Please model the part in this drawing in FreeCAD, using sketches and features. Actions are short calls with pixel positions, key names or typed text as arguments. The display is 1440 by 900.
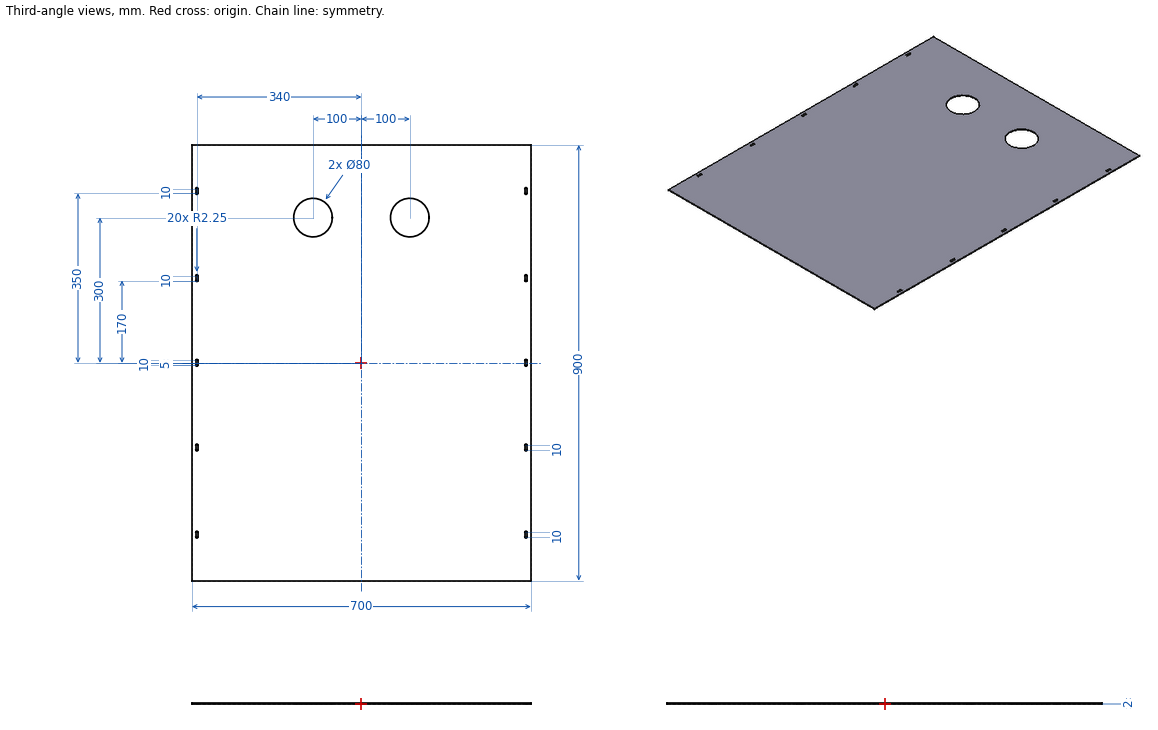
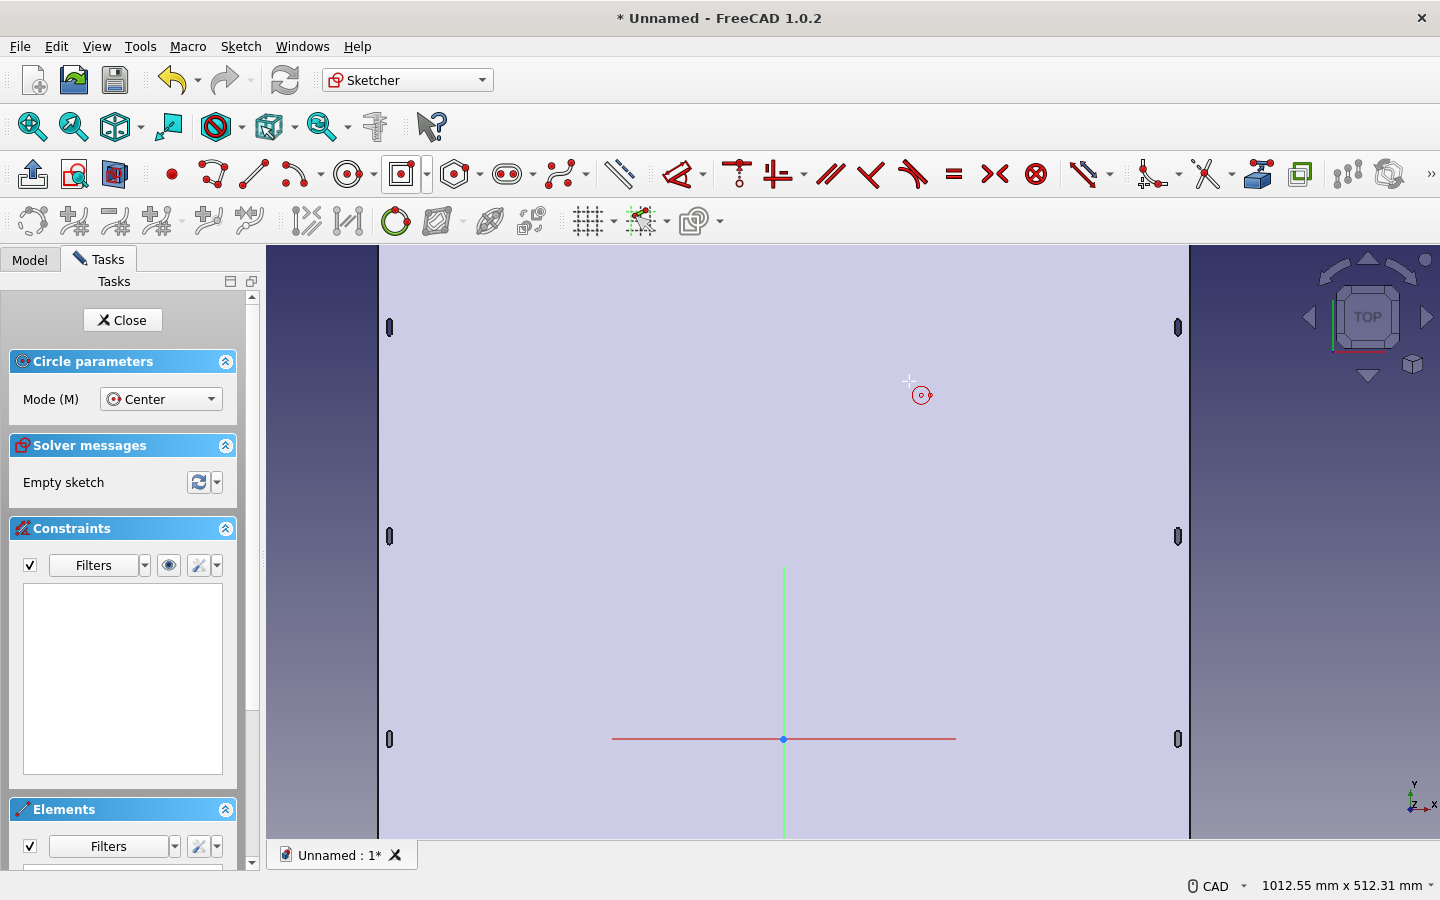
click(668, 391)
click(701, 358)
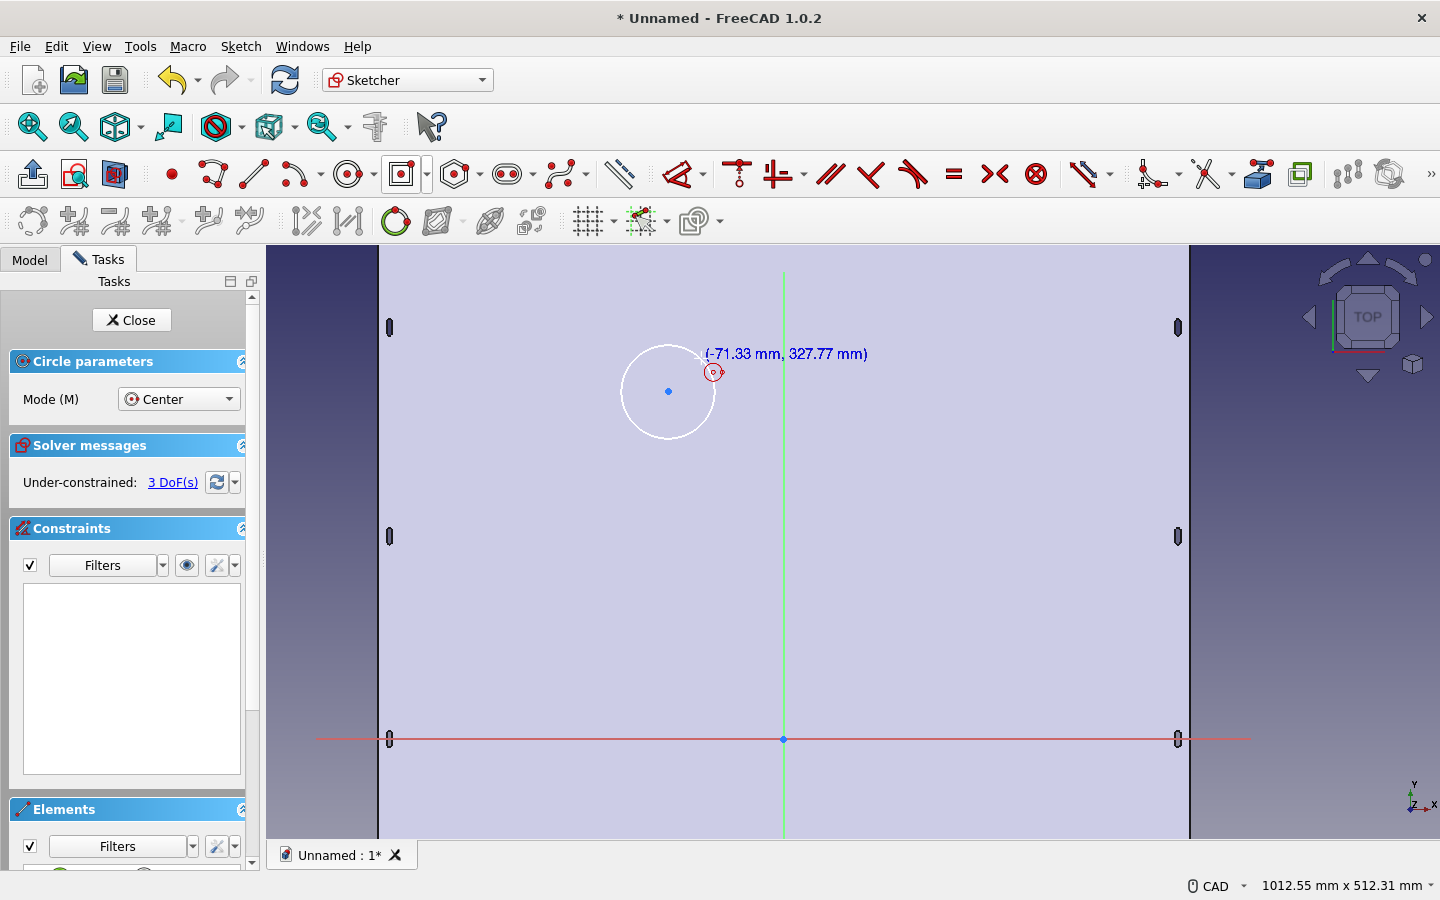
click(900, 391)
click(932, 358)
key(Escape)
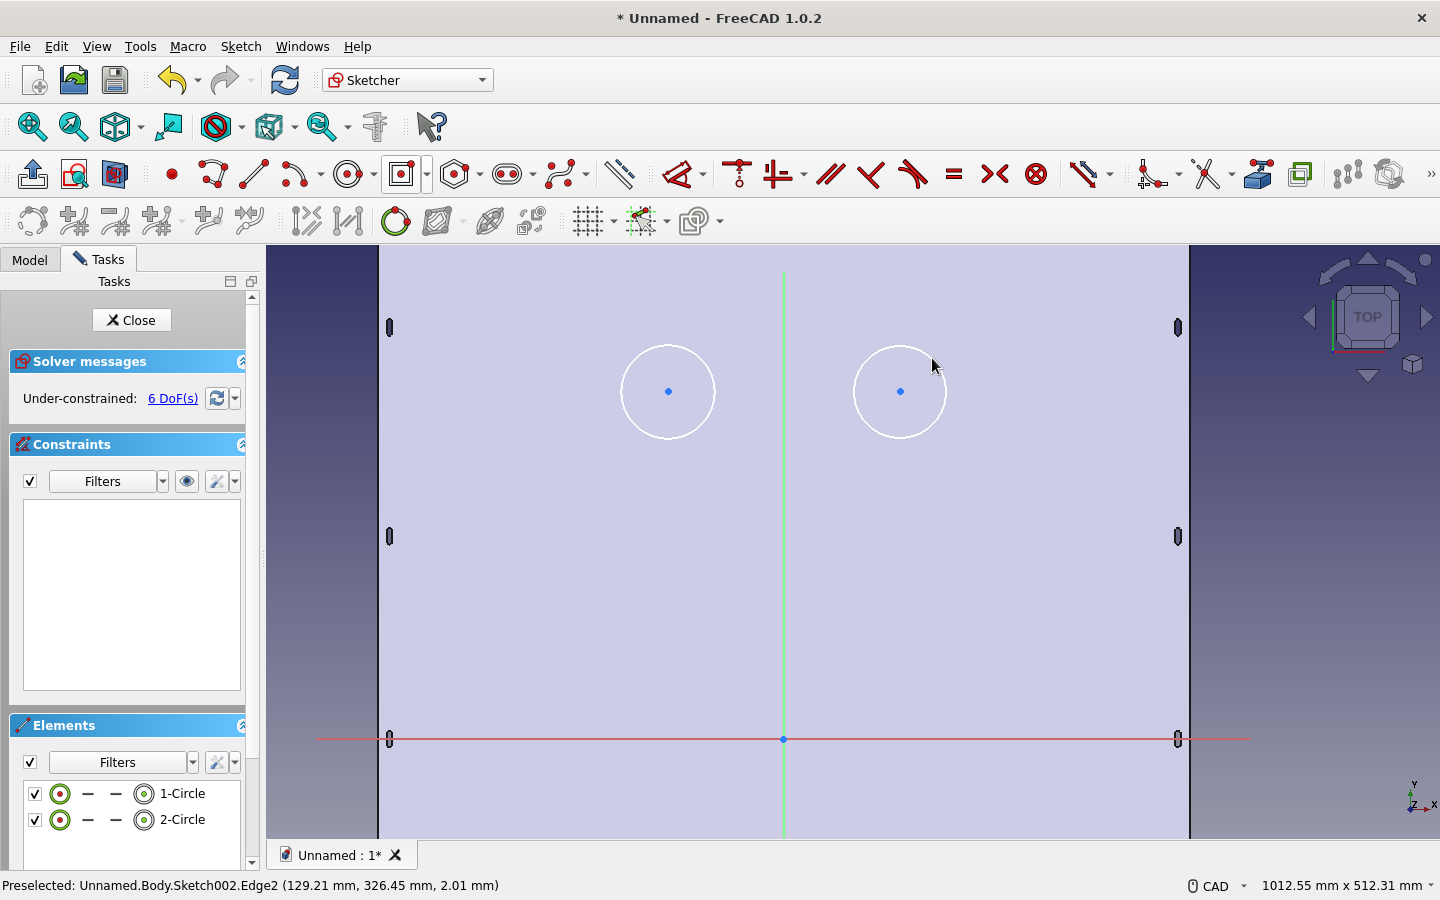
click(701, 359)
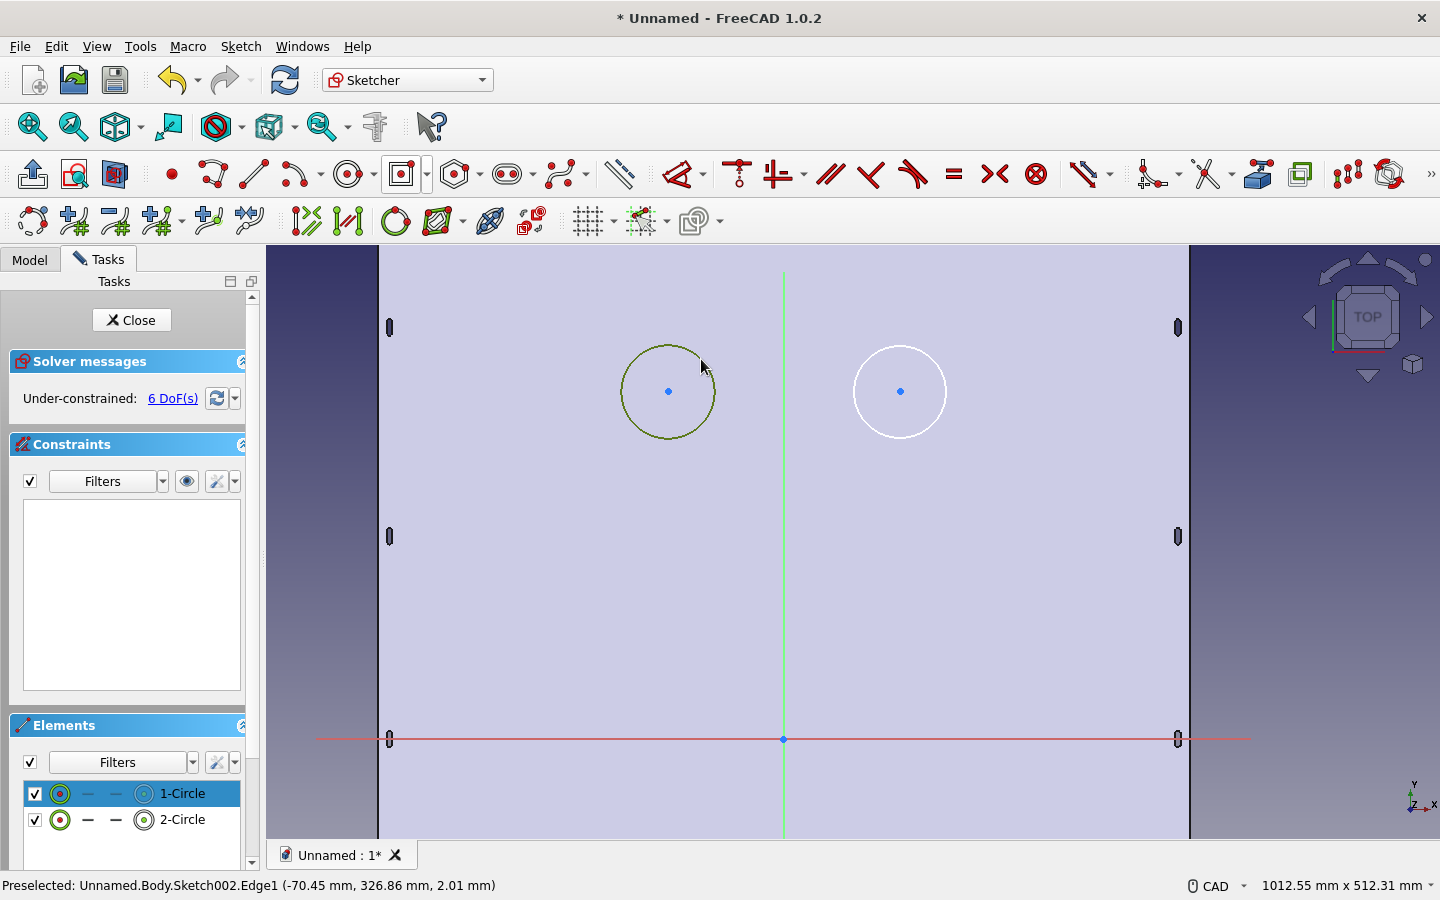
click(932, 359)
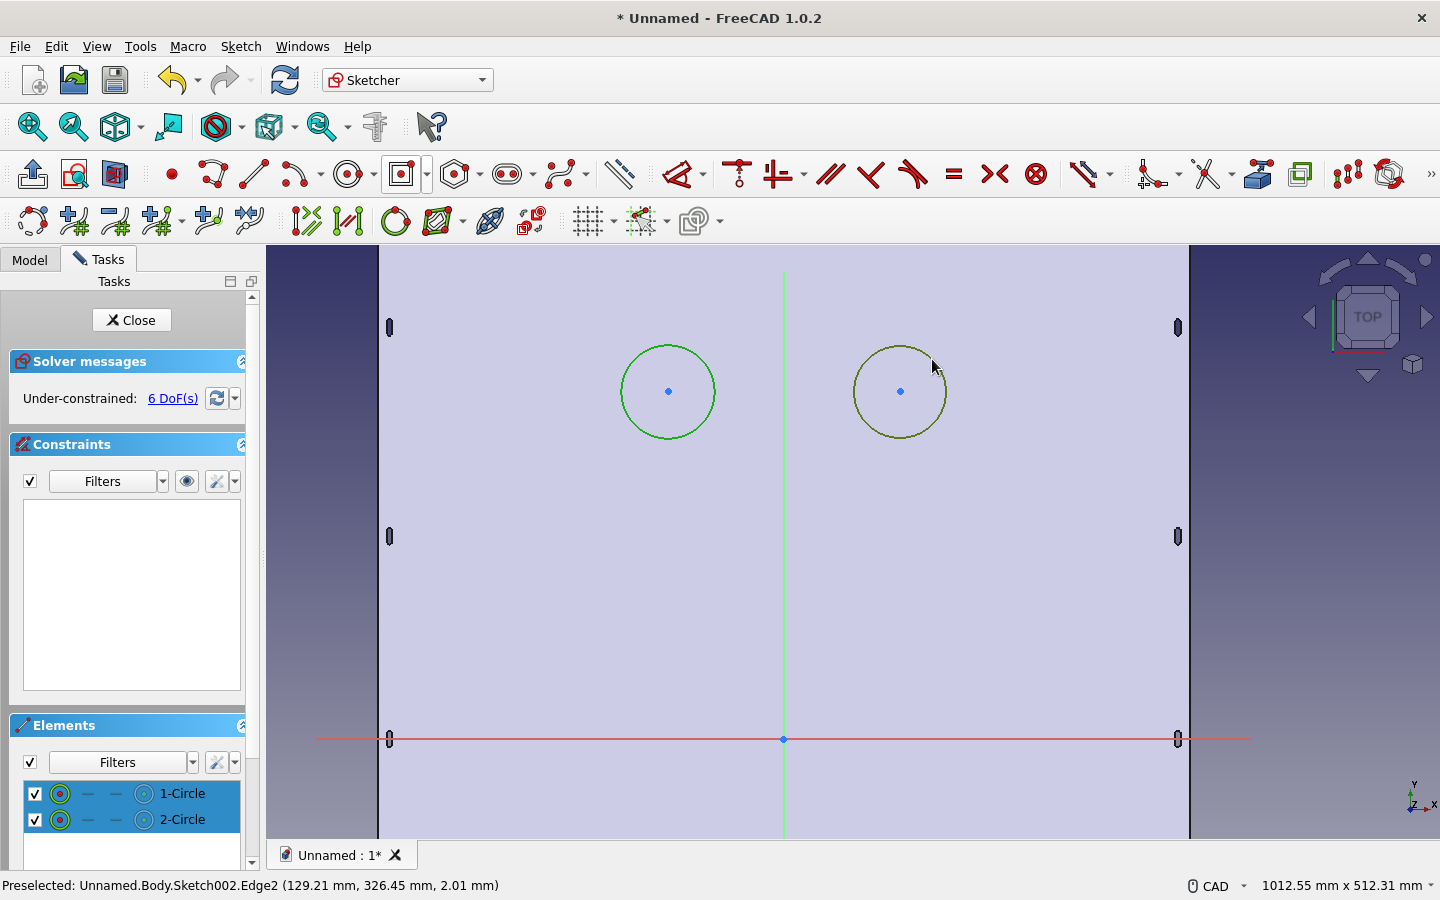
click(954, 174)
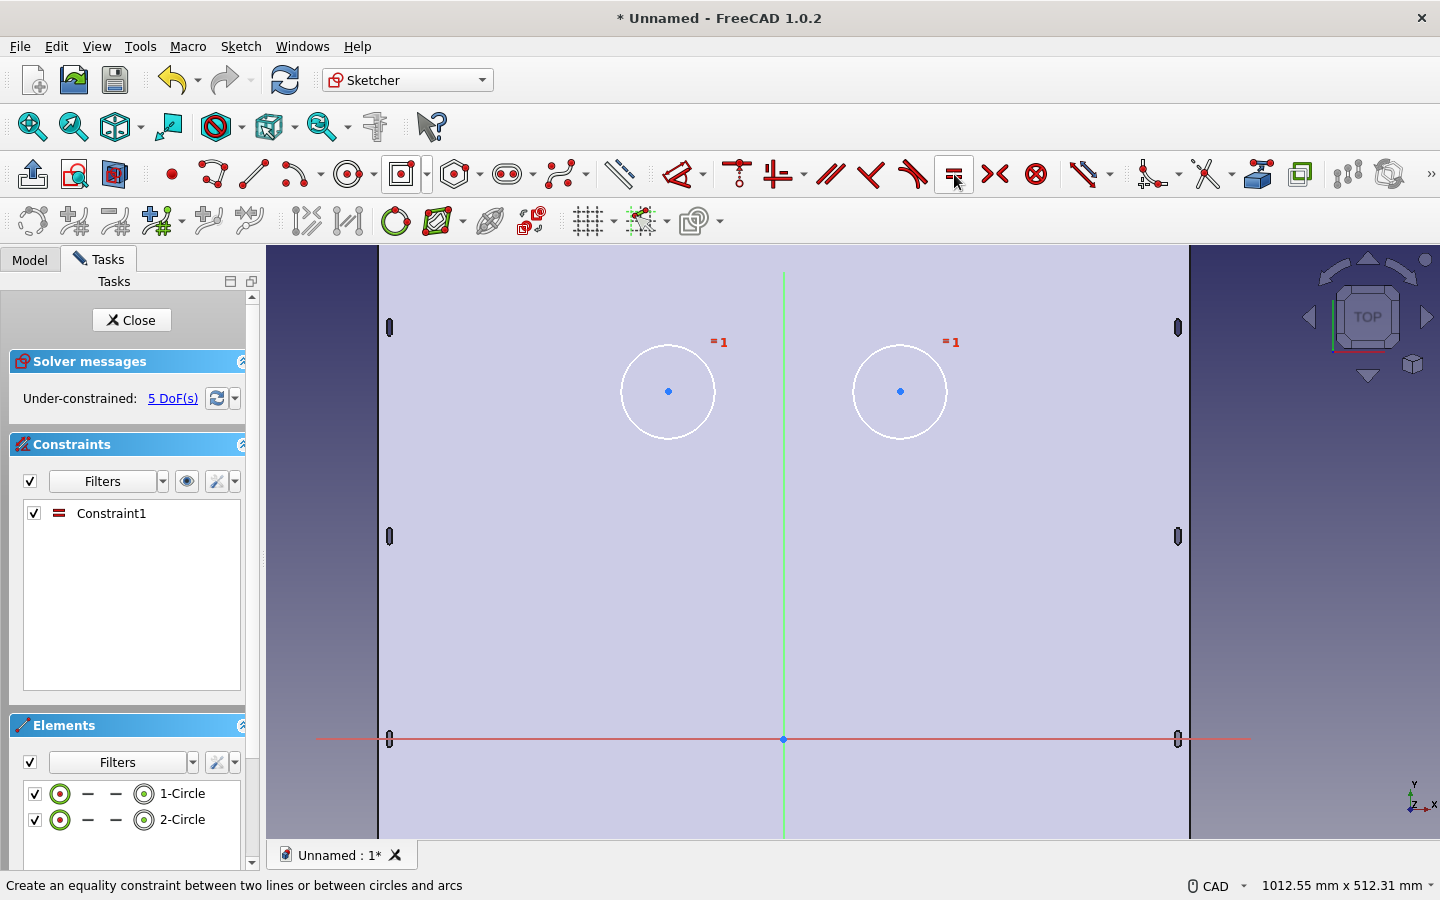
click(668, 392)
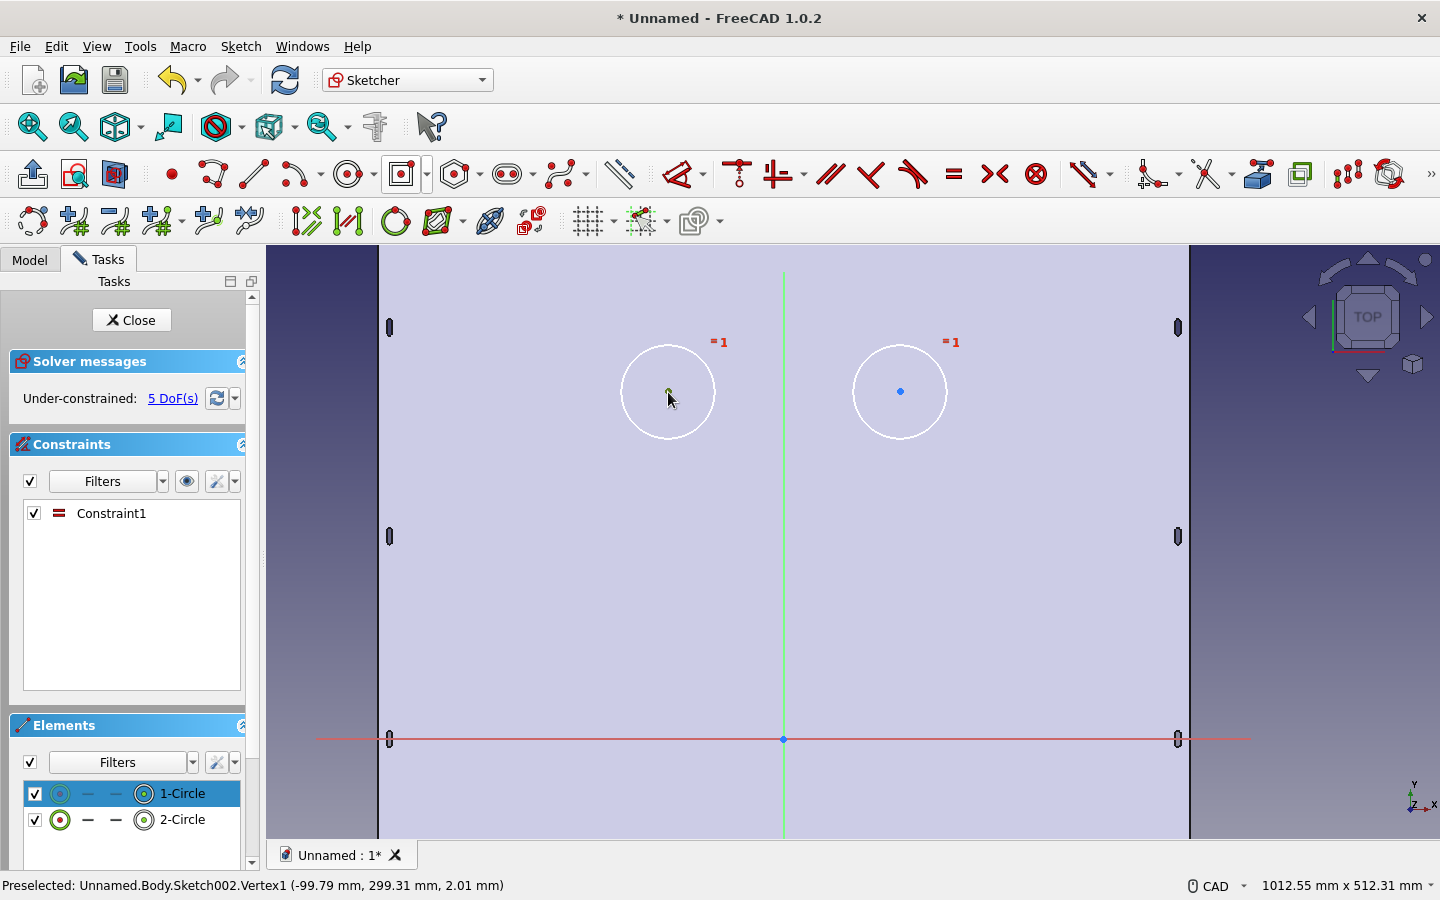
click(900, 392)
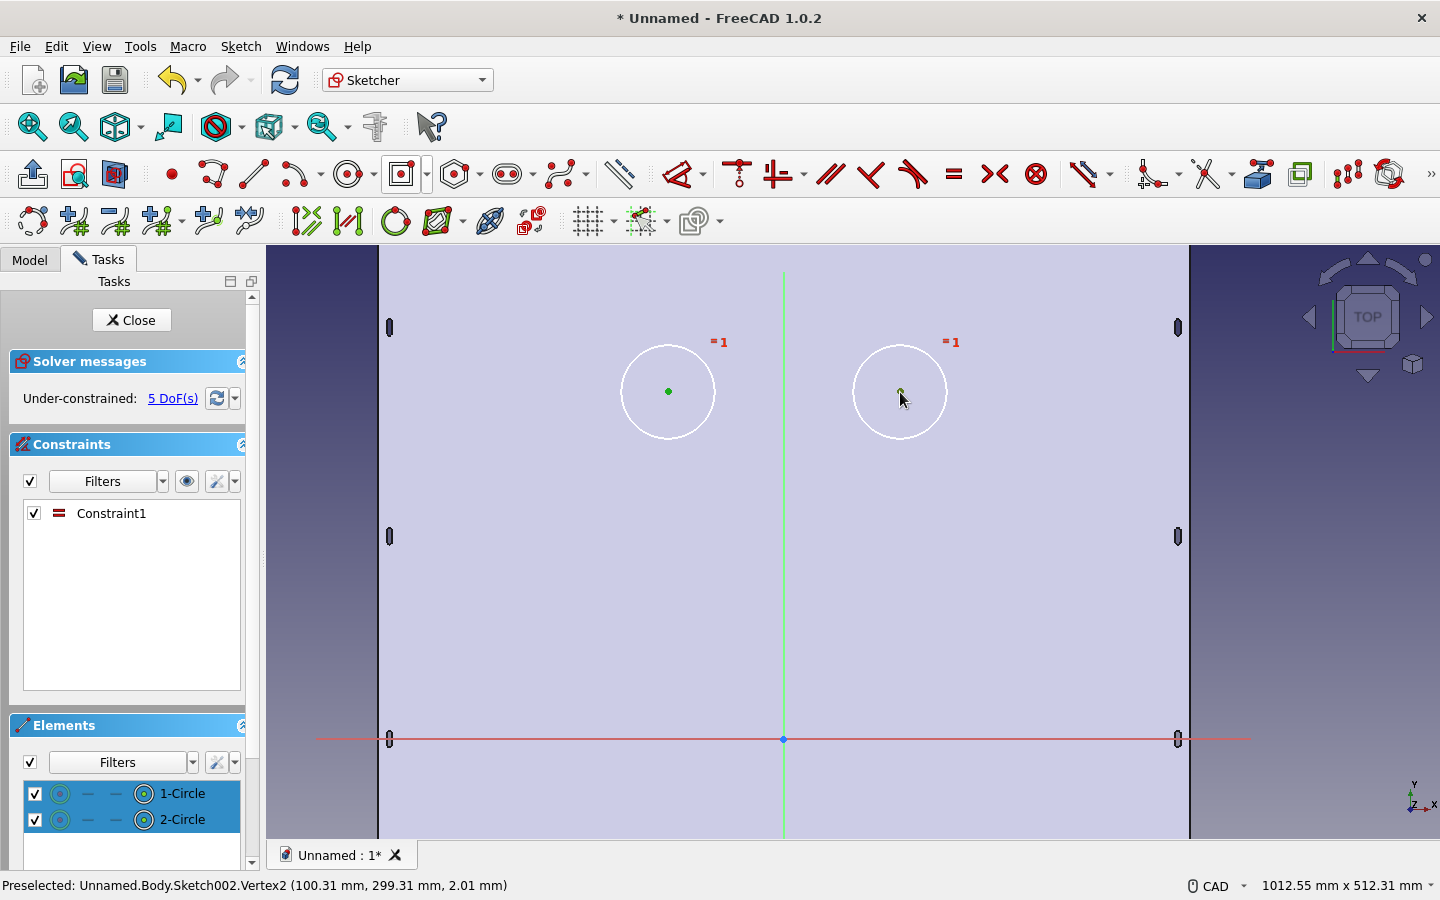
key(h)